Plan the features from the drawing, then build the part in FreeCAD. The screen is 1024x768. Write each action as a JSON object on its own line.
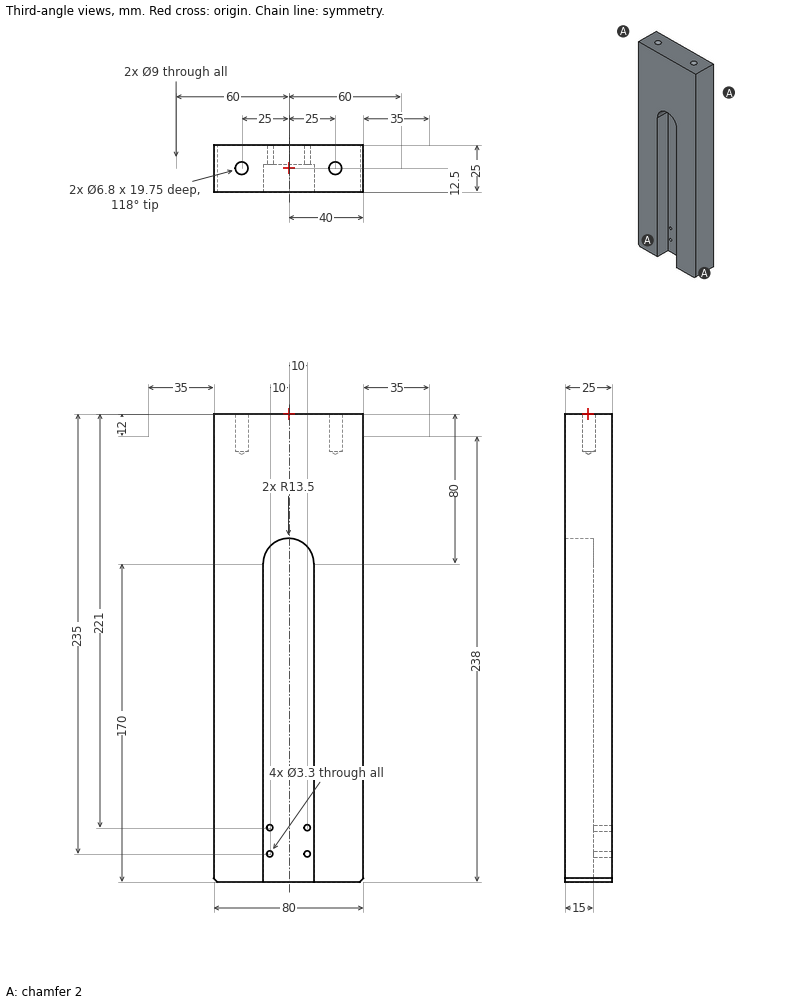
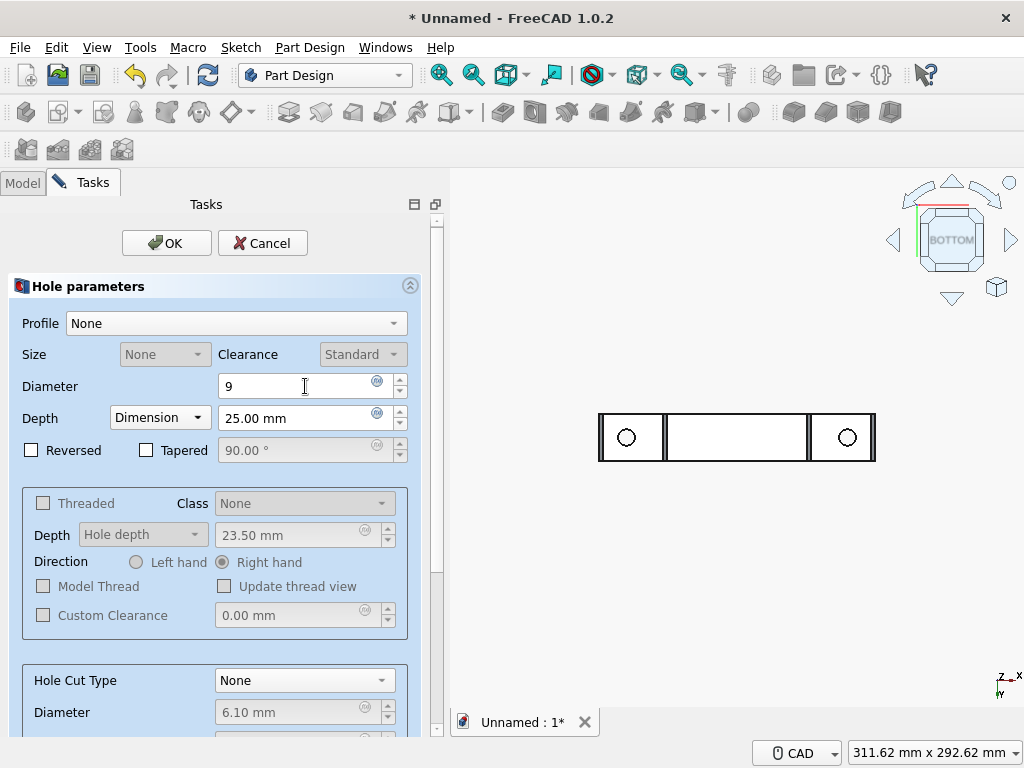
{"action": "left_click", "coordinate": [161, 418]}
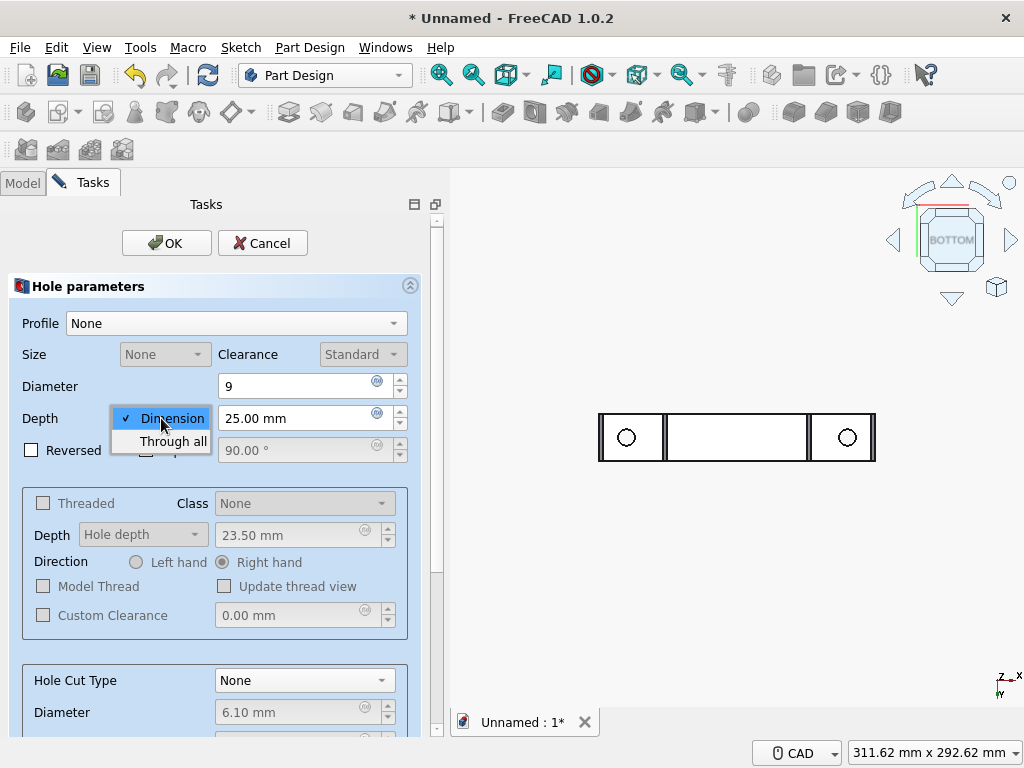
{"action": "left_click", "coordinate": [160, 442]}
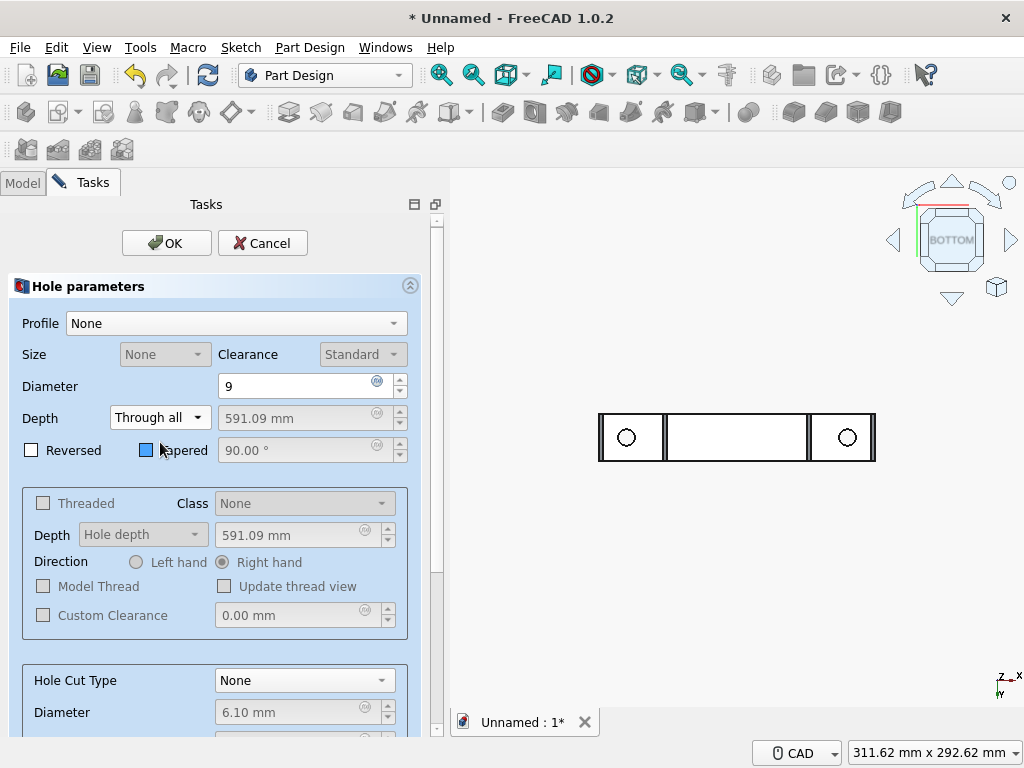
{"action": "left_click", "coordinate": [167, 243]}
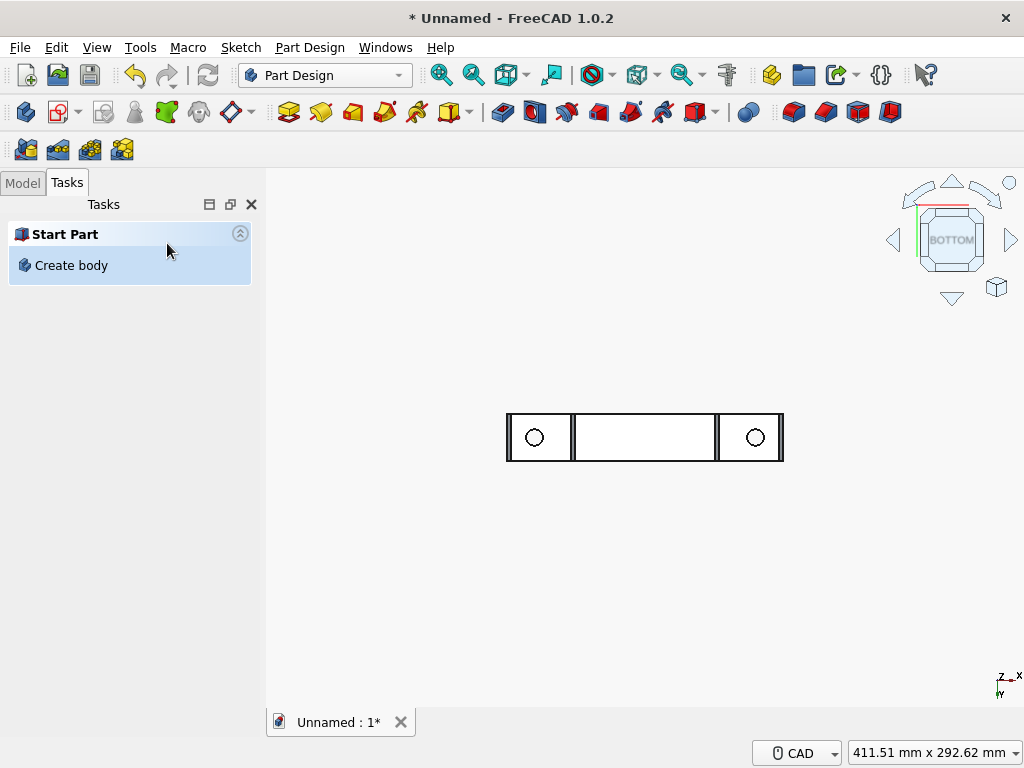
{"action": "left_click", "coordinate": [442, 76]}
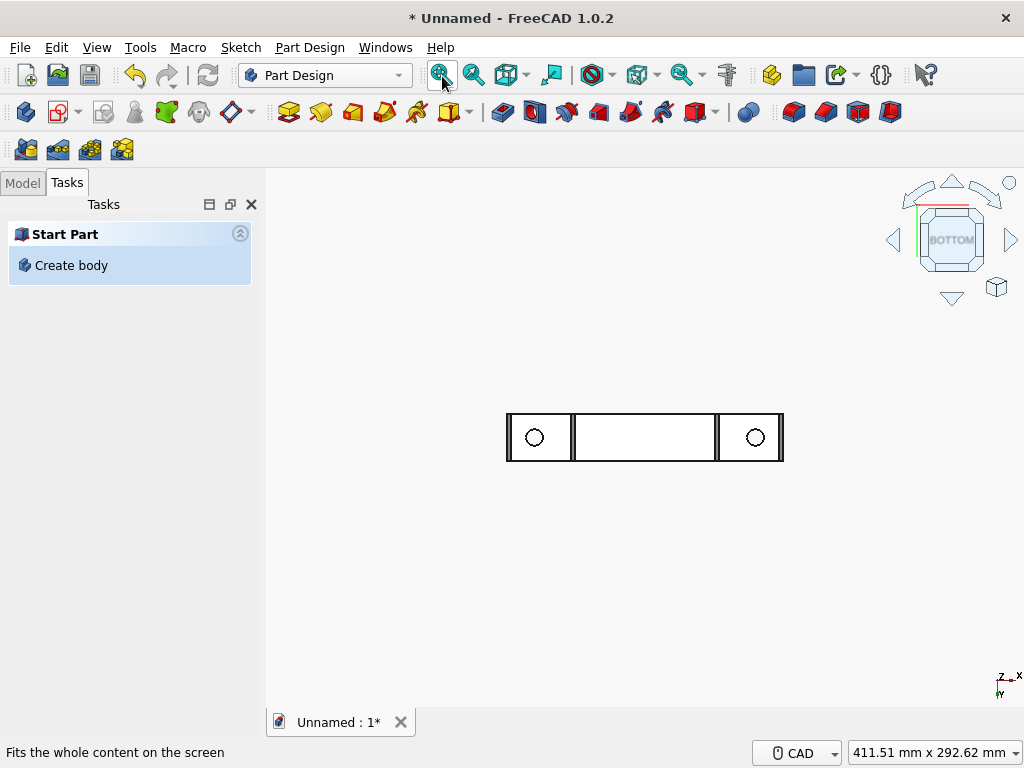
{"action": "key", "text": "0"}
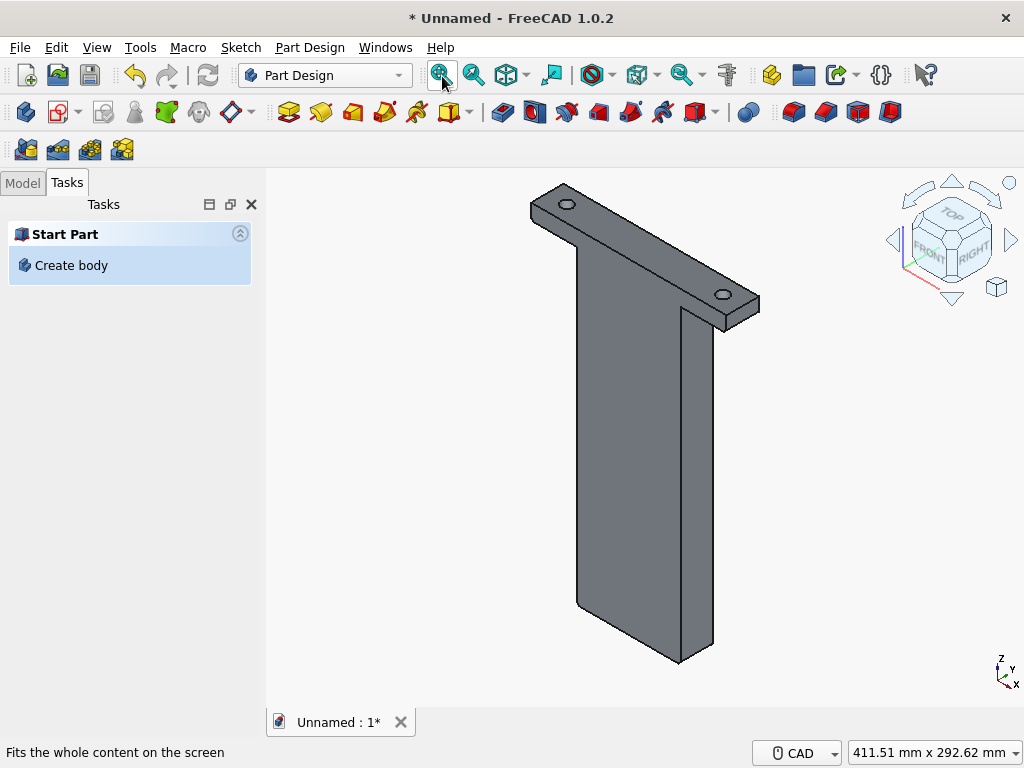
{"action": "left_click", "coordinate": [629, 338]}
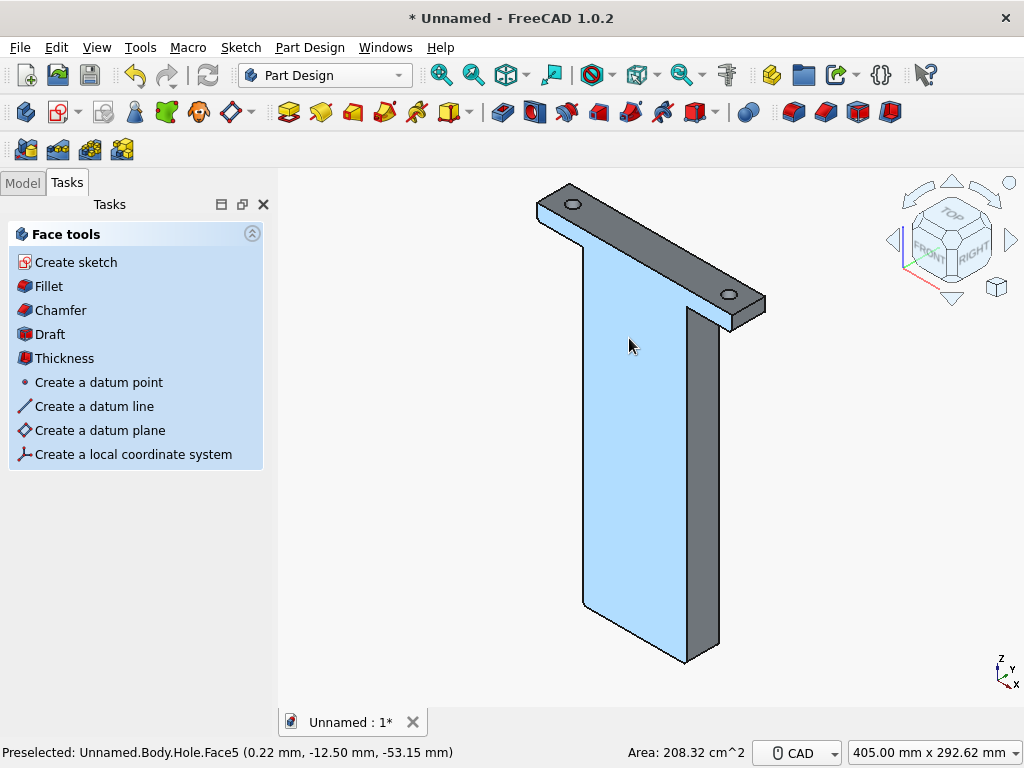
{"action": "left_click", "coordinate": [58, 112]}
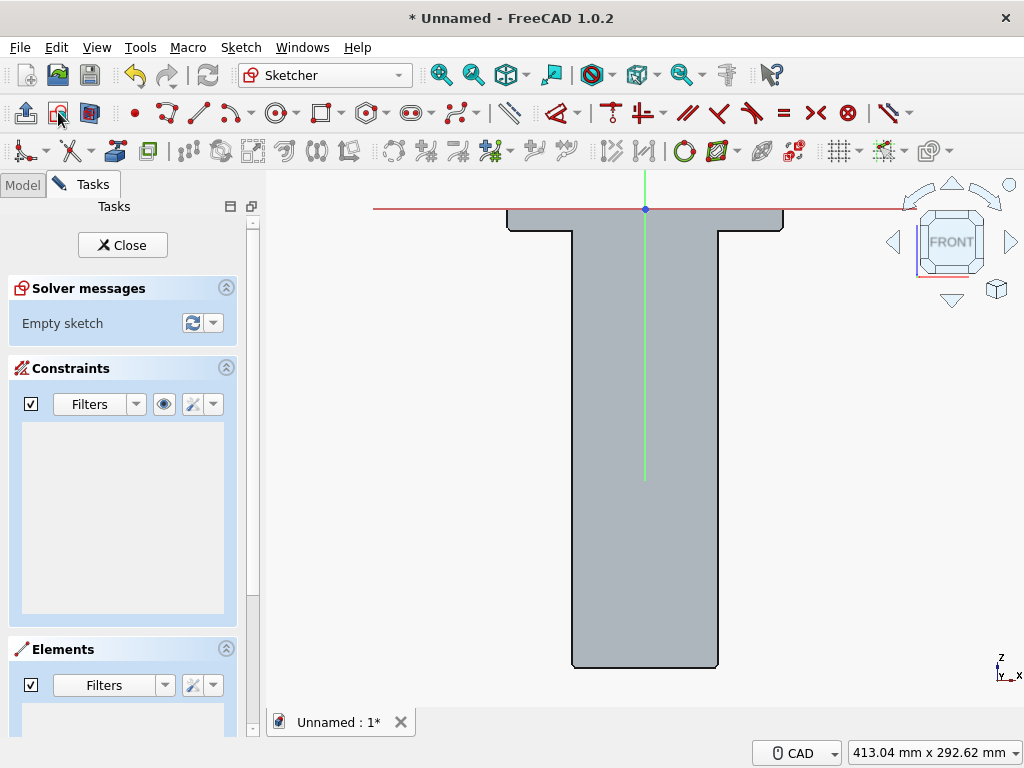
{"action": "scroll", "coordinate": [437, 413], "scroll_direction": "down", "scroll_amount": 2}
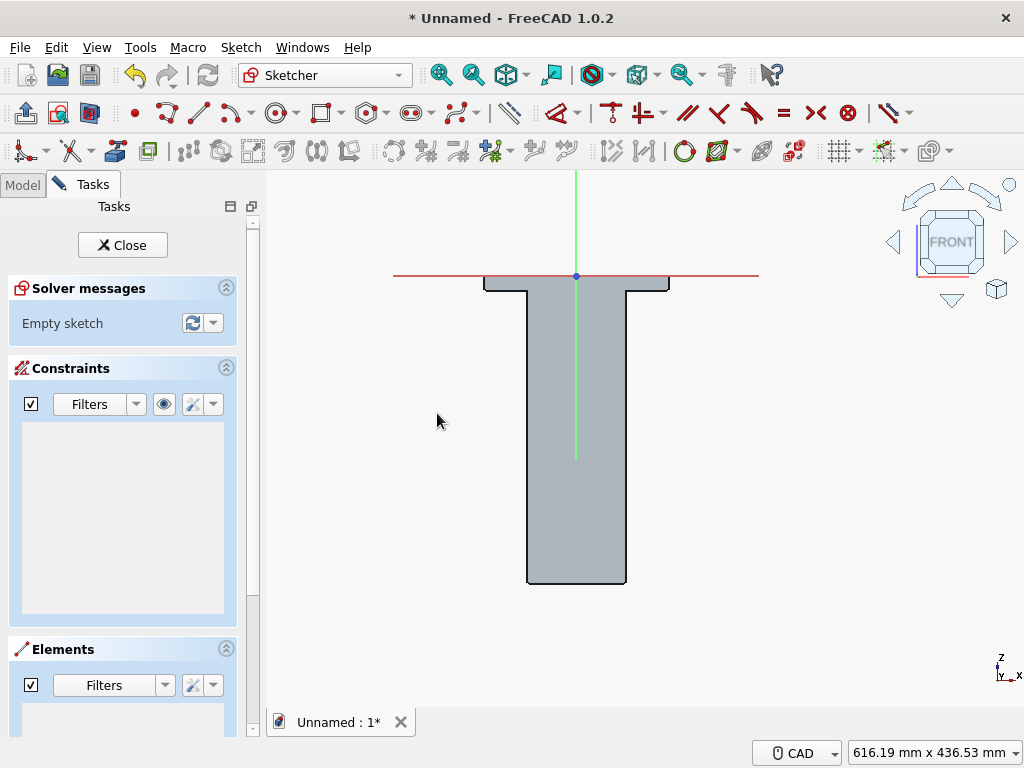
{"action": "left_click", "coordinate": [412, 114]}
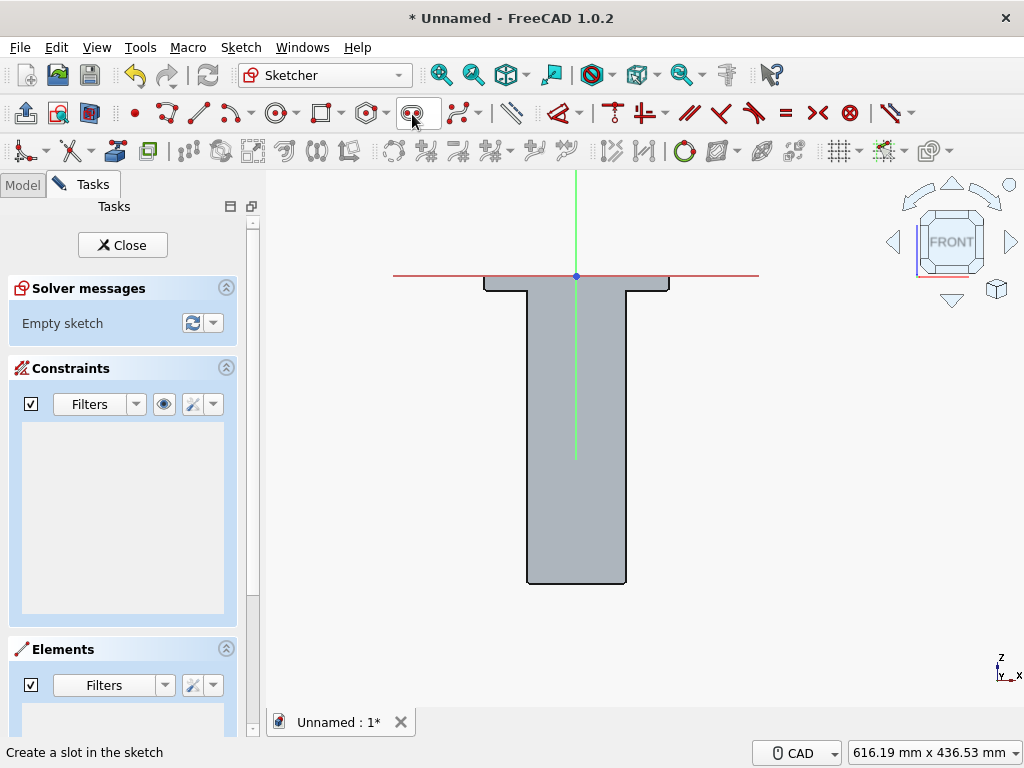
{"action": "scroll", "coordinate": [577, 584], "scroll_direction": "up", "scroll_amount": 2}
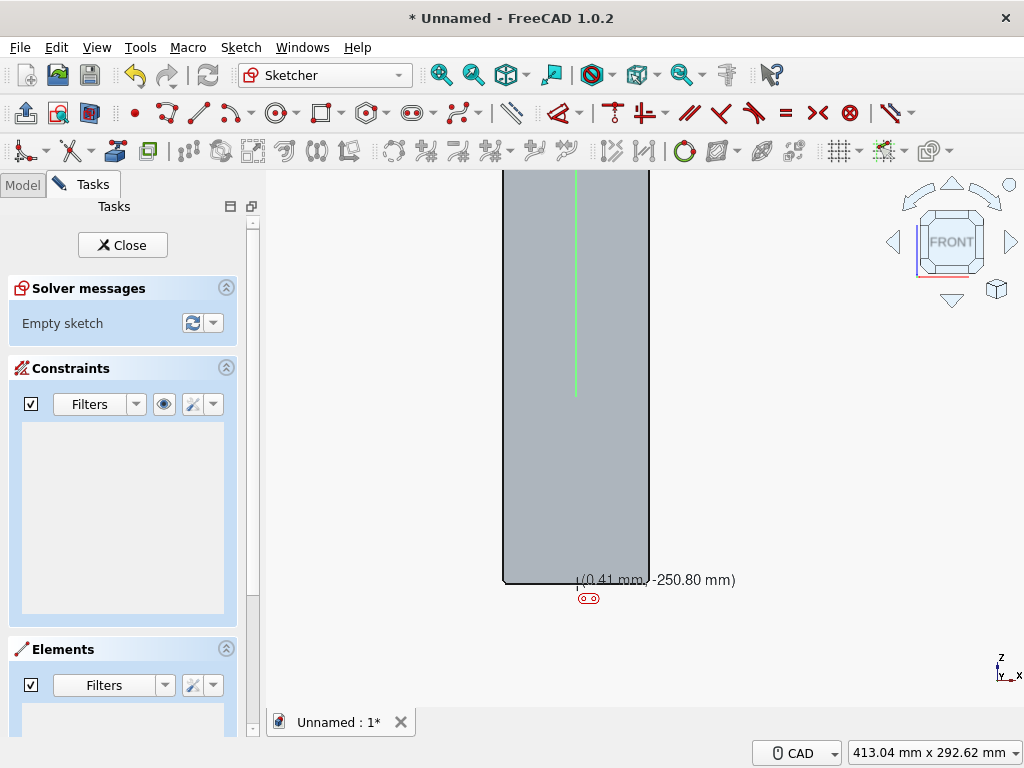
{"action": "left_click", "coordinate": [576, 584]}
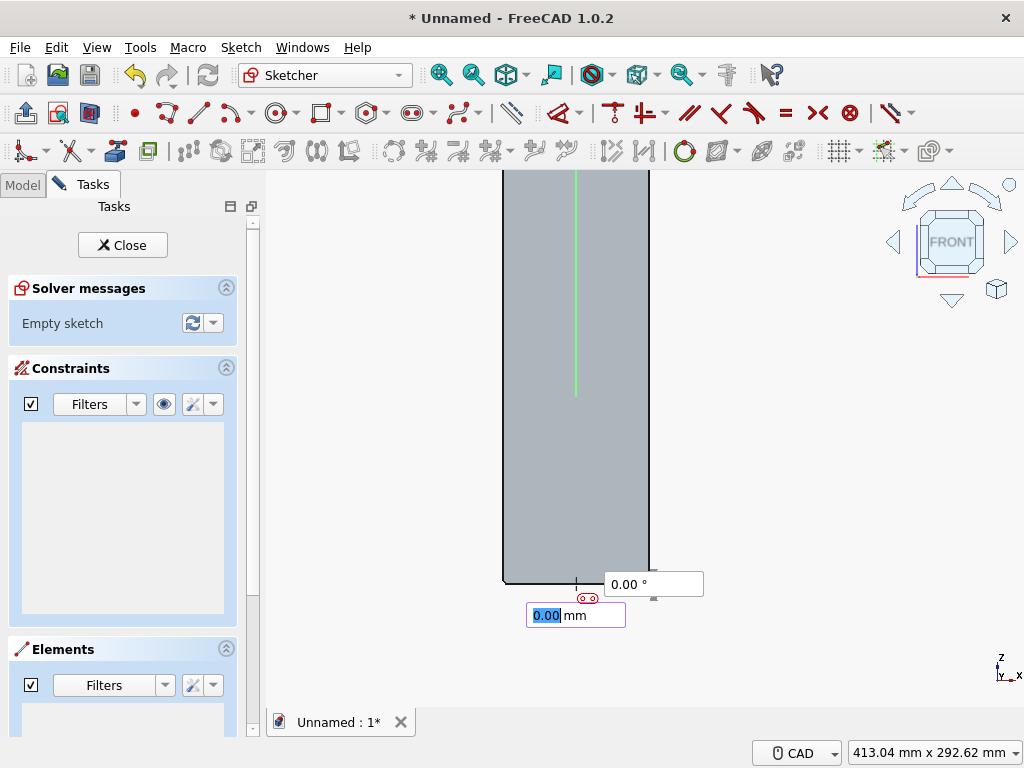
{"action": "left_click", "coordinate": [585, 272]}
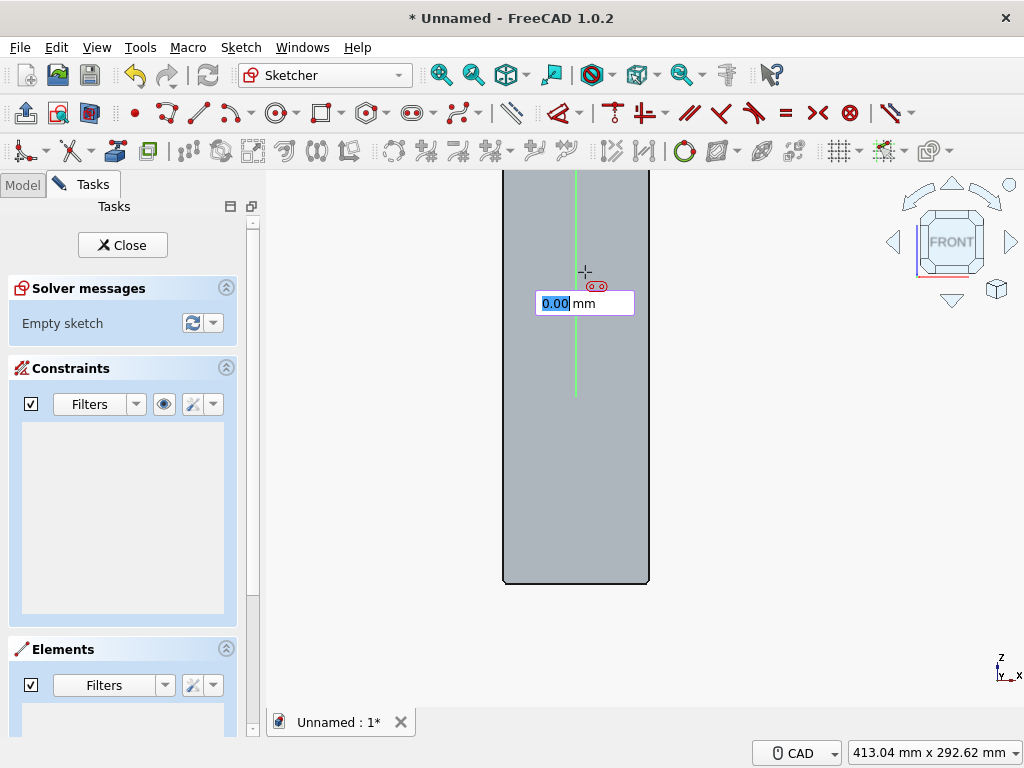
{"action": "left_click", "coordinate": [601, 428]}
{"action": "key", "text": "Escape"}